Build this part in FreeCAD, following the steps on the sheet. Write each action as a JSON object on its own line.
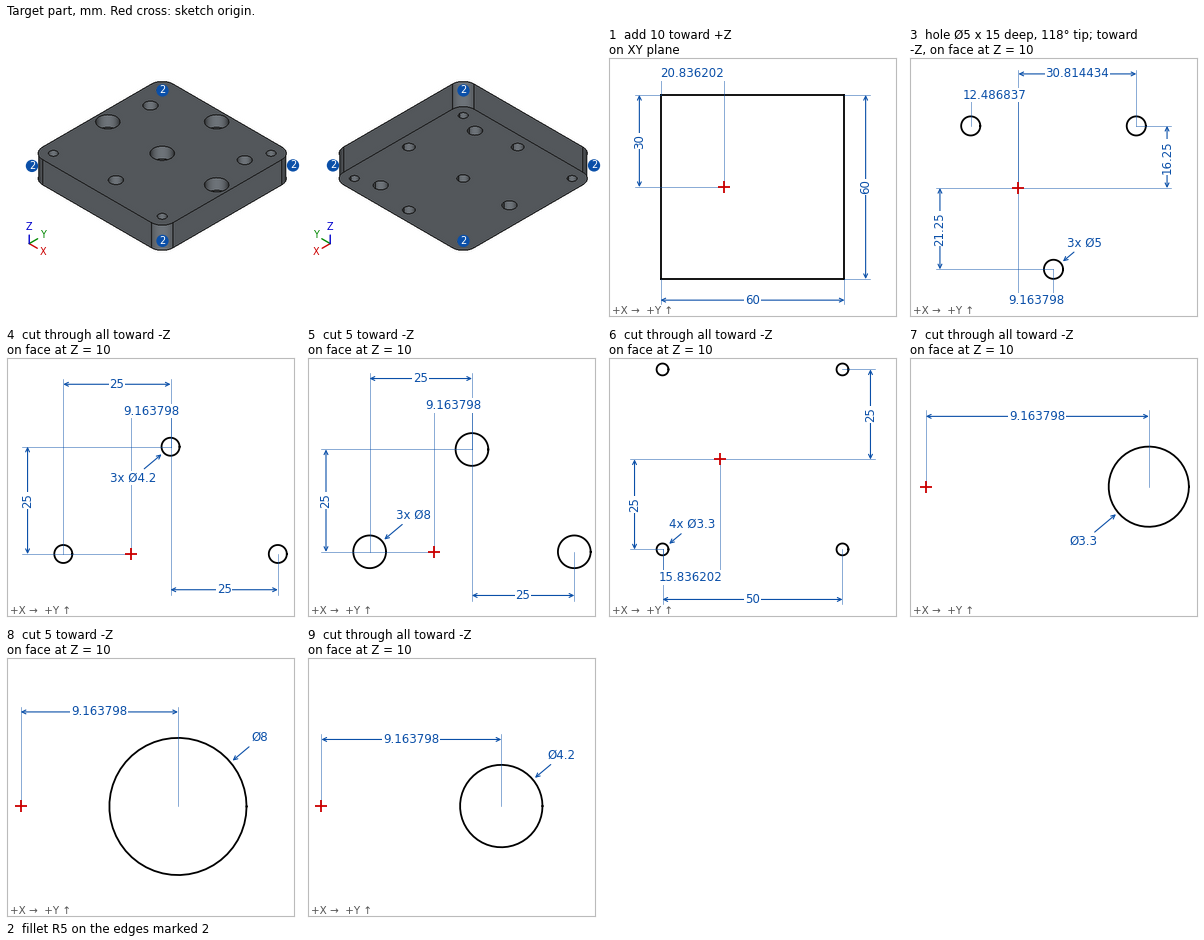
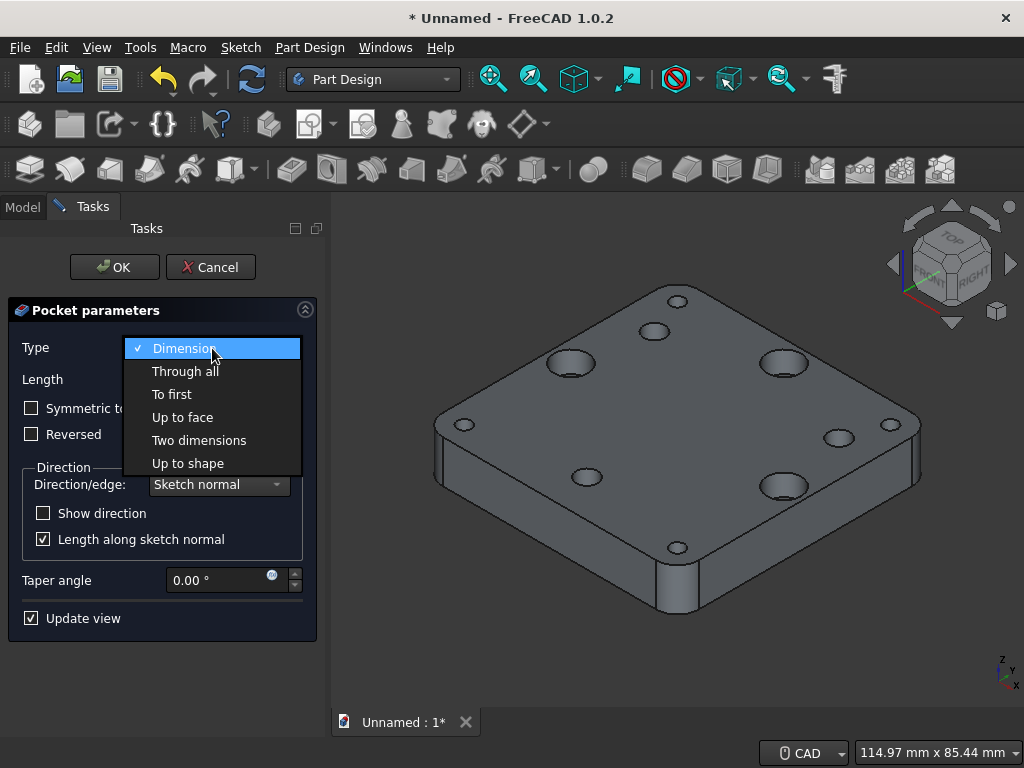
{"action": "left_click", "coordinate": [212, 372]}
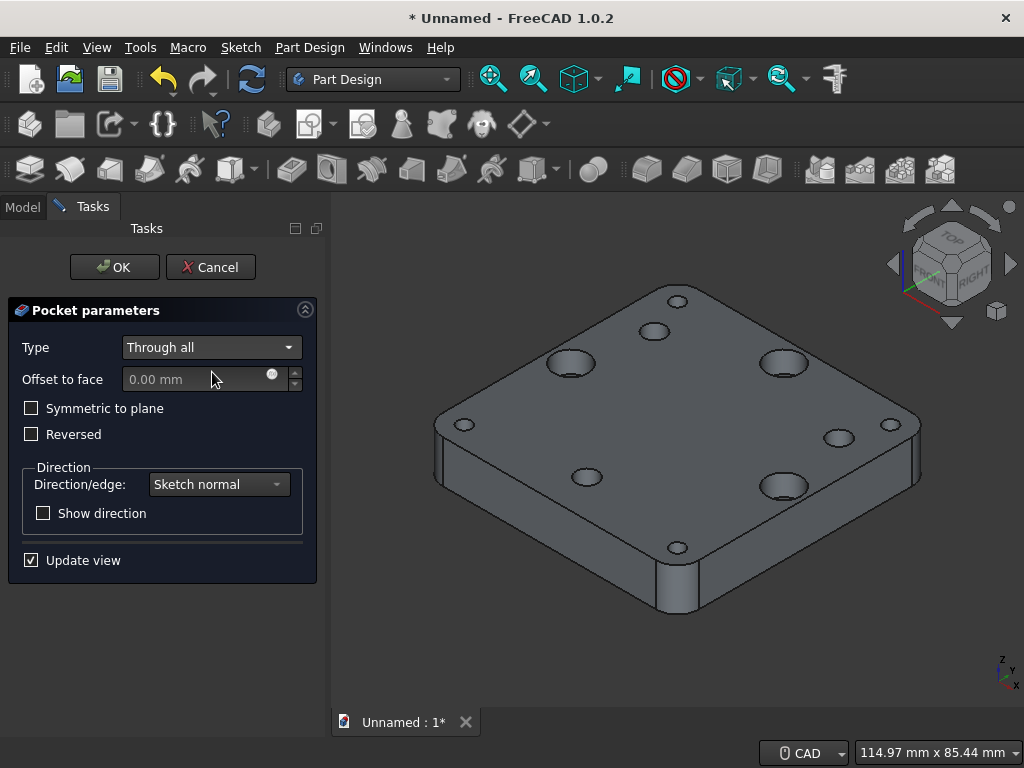
{"action": "left_click", "coordinate": [115, 267]}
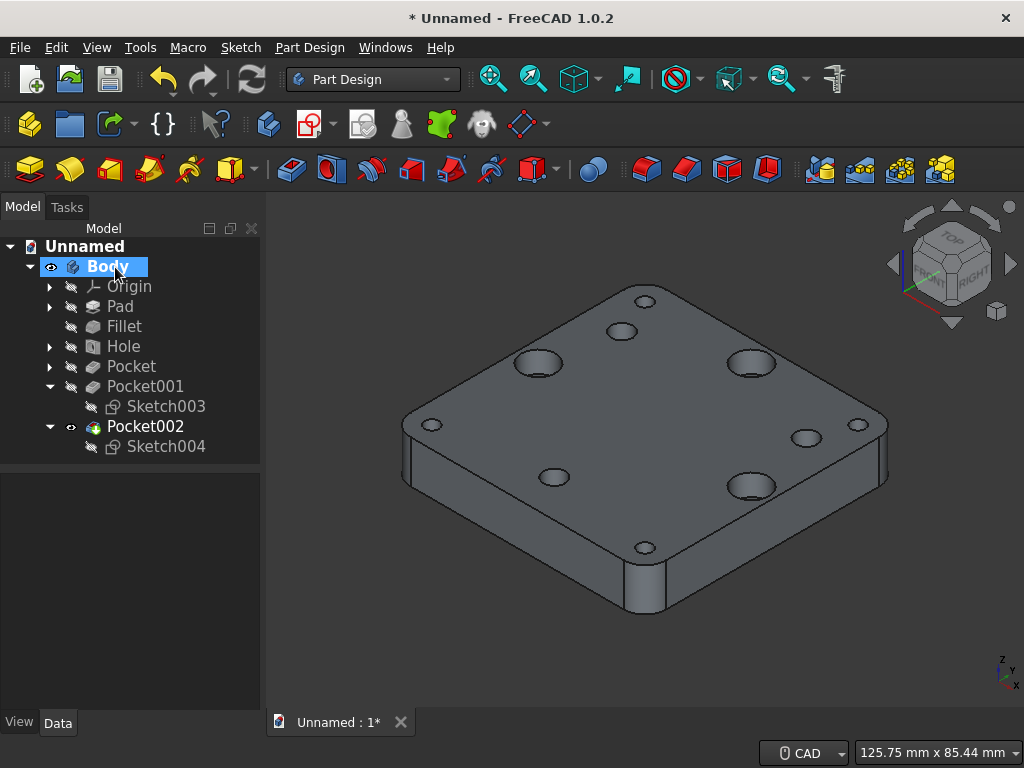
{"action": "left_click", "coordinate": [645, 424]}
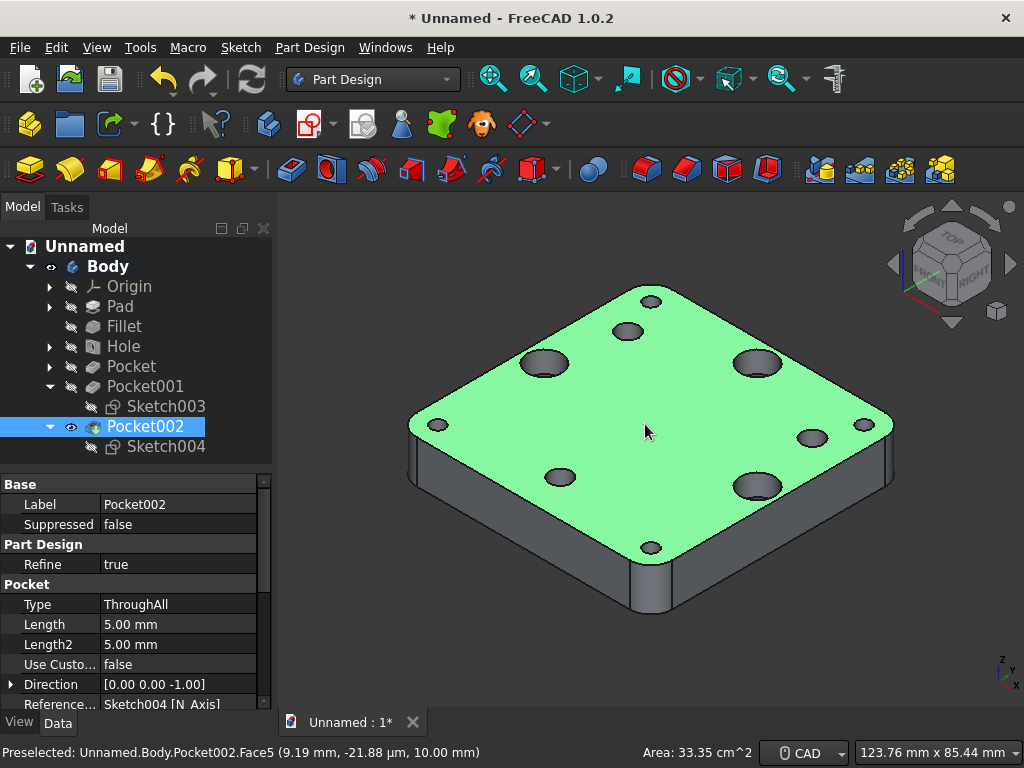
{"action": "left_click", "coordinate": [310, 124]}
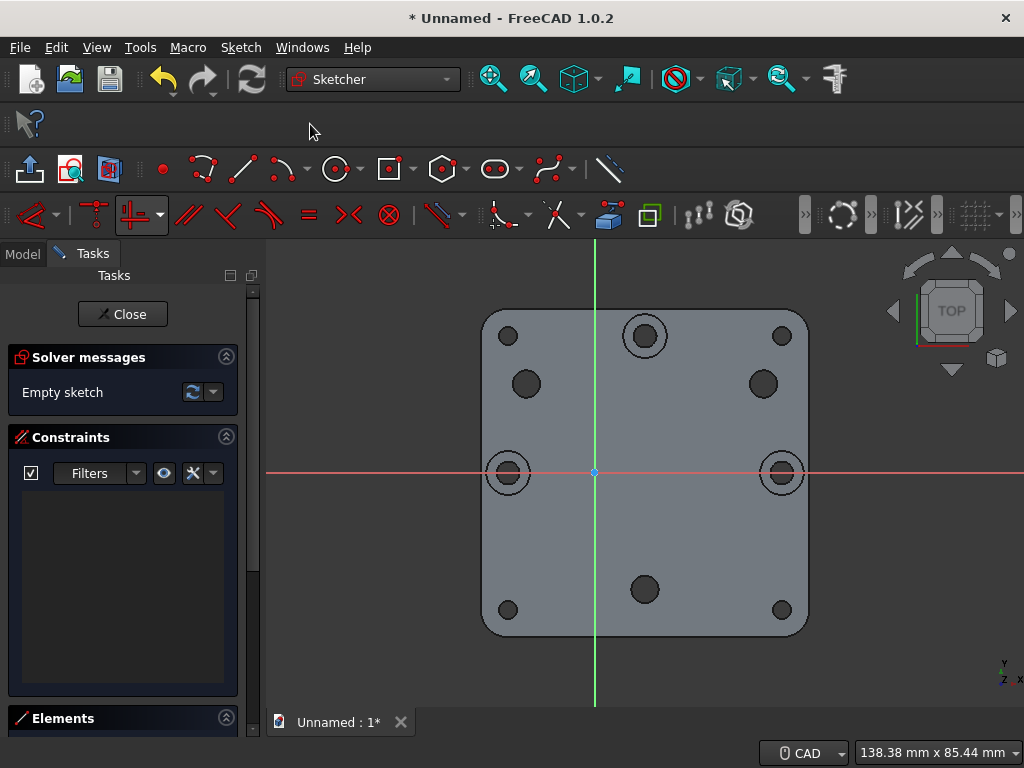
{"action": "scroll", "coordinate": [649, 473], "scroll_direction": "up", "scroll_amount": 14}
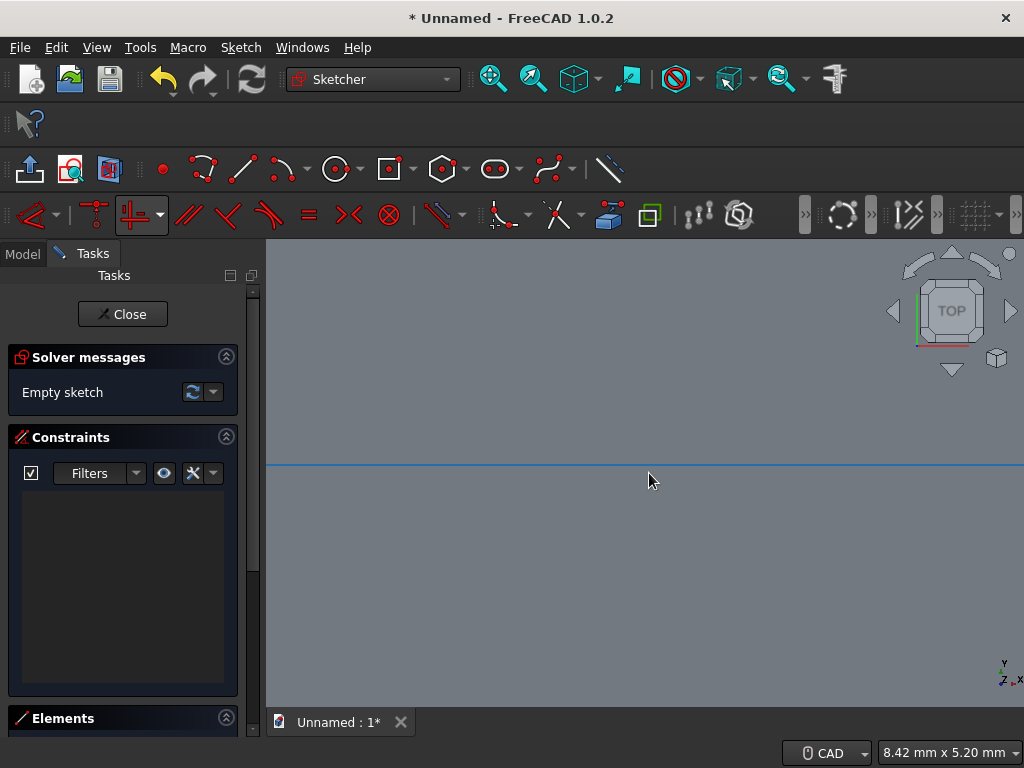
{"action": "left_click", "coordinate": [336, 170]}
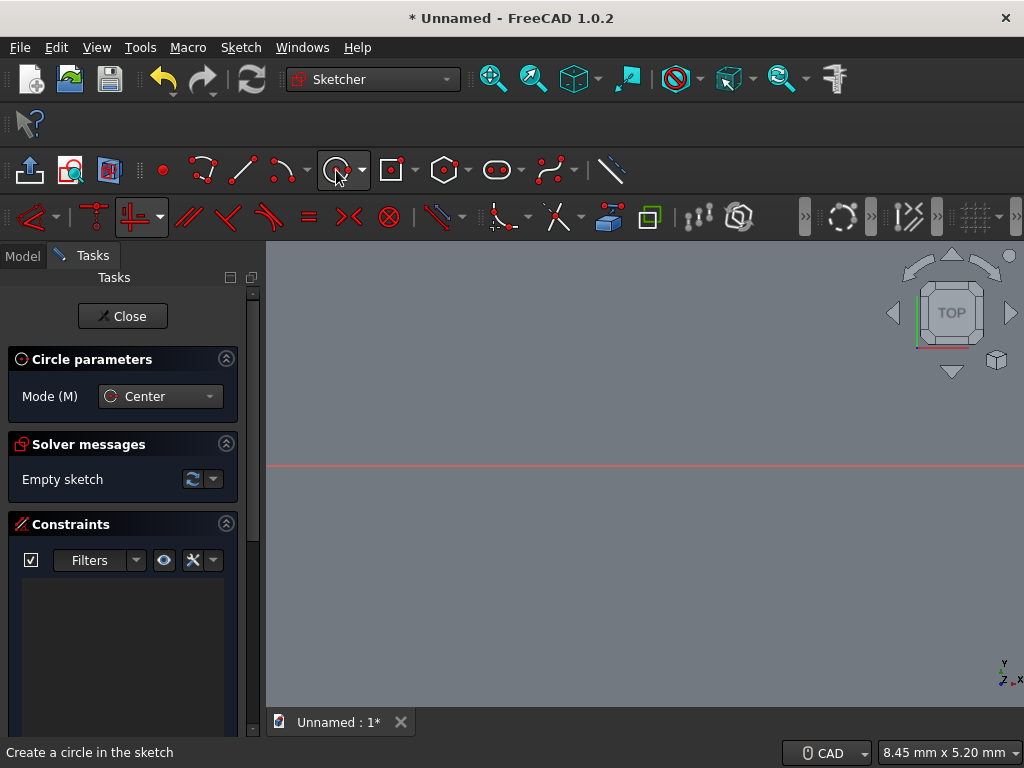
{"action": "left_click", "coordinate": [576, 466]}
{"action": "mouse_move", "coordinate": [680, 362]}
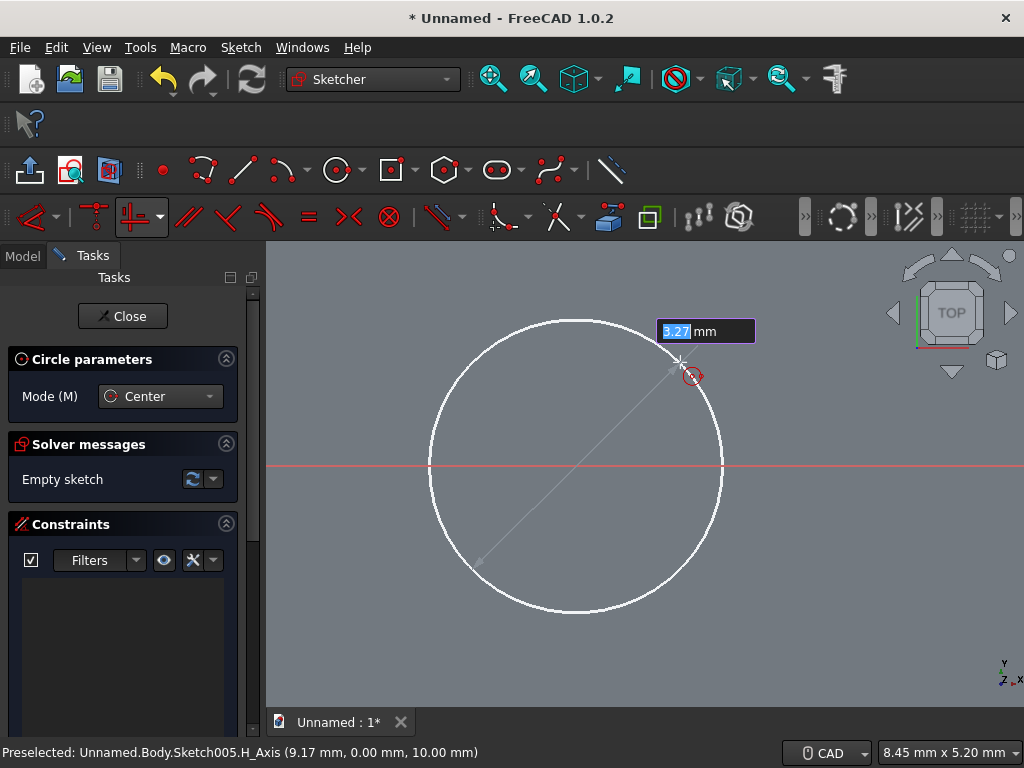
{"action": "type", "text": "3.3"}
{"action": "key", "text": "Return"}
{"action": "key", "text": "Escape"}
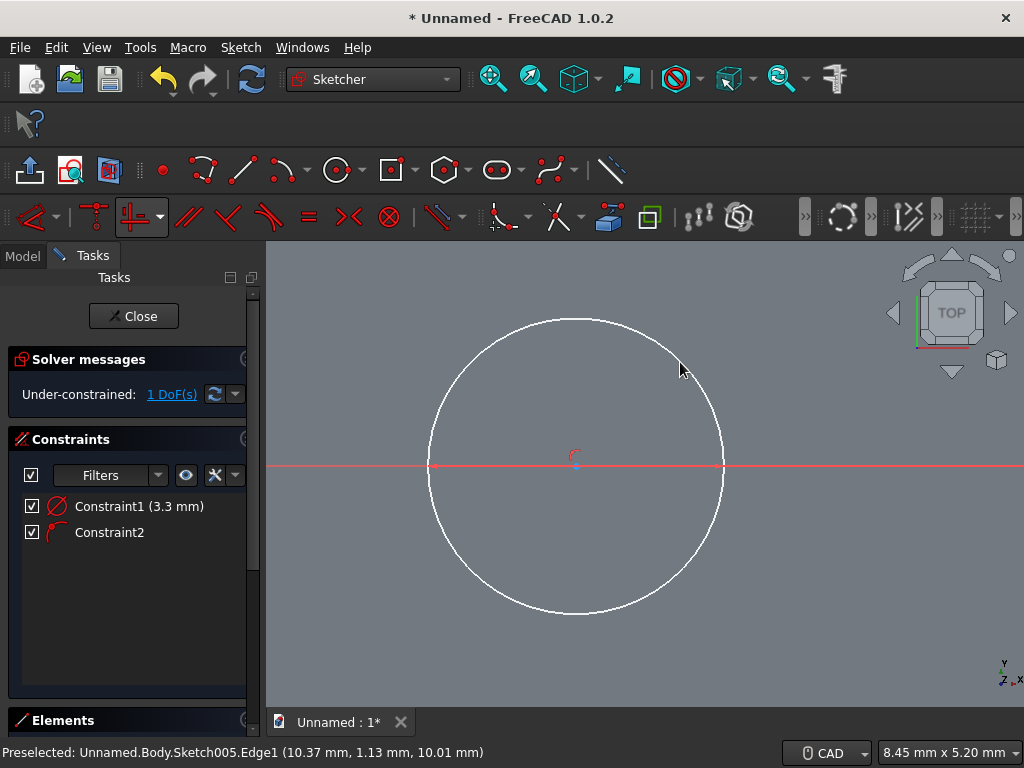
{"action": "left_click", "coordinate": [32, 218]}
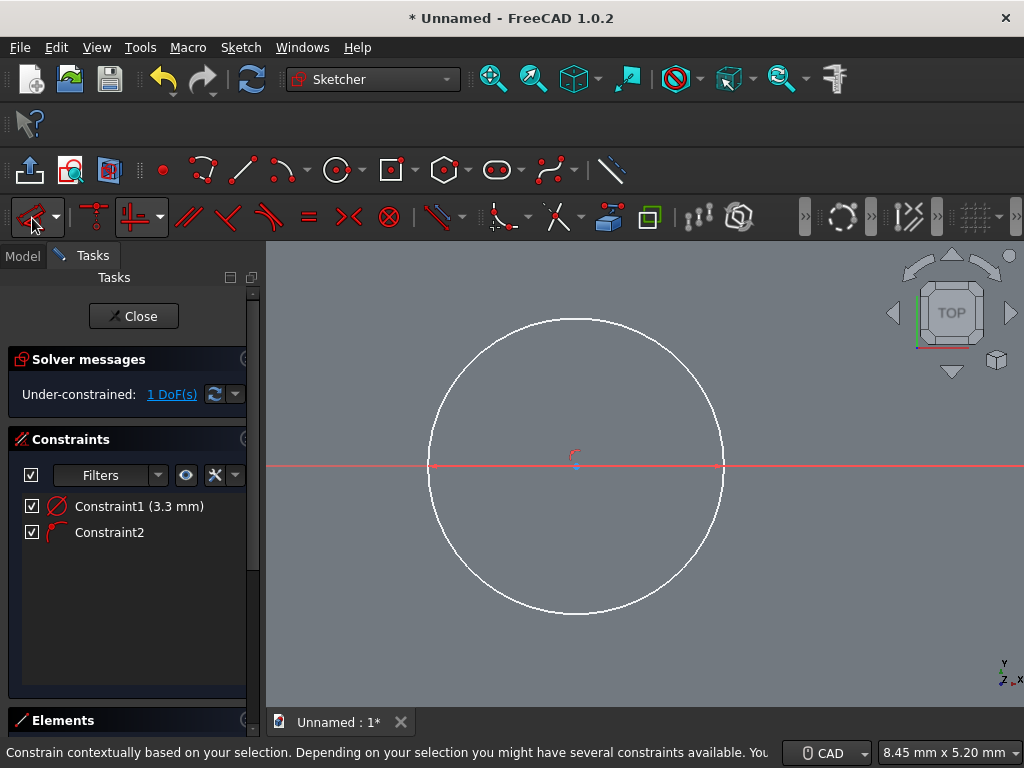
{"action": "left_click", "coordinate": [576, 466]}
{"action": "left_click", "coordinate": [370, 500]}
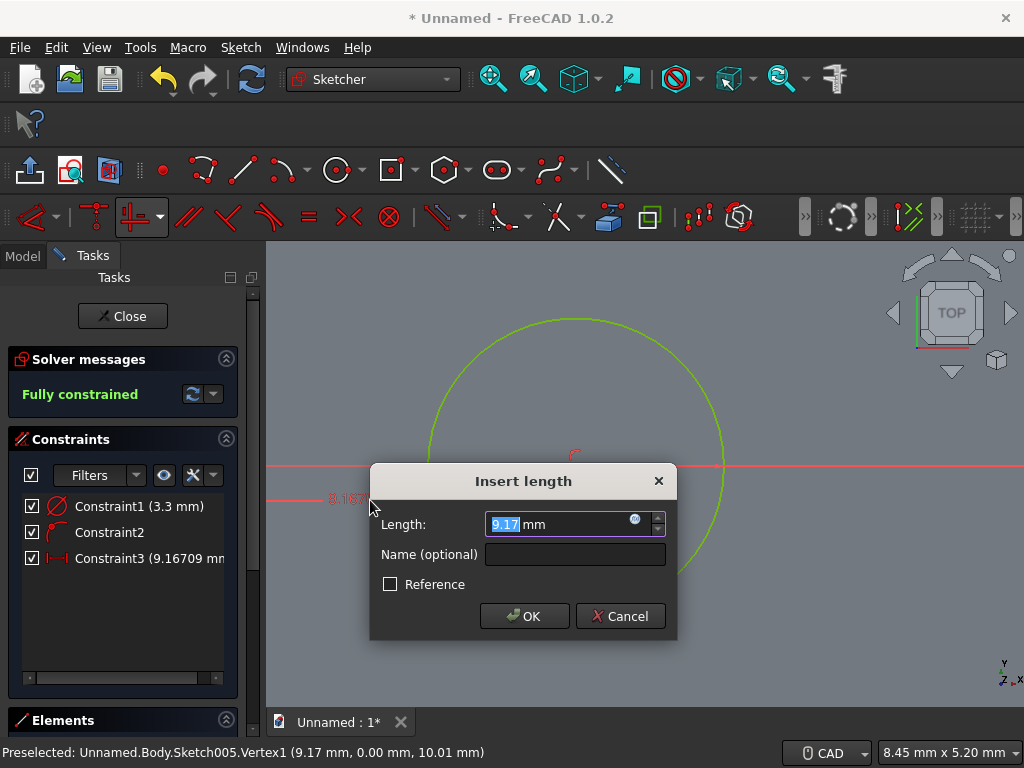
{"action": "type", "text": "9.163798"}
{"action": "key", "text": "Return"}
{"action": "key", "text": "Escape"}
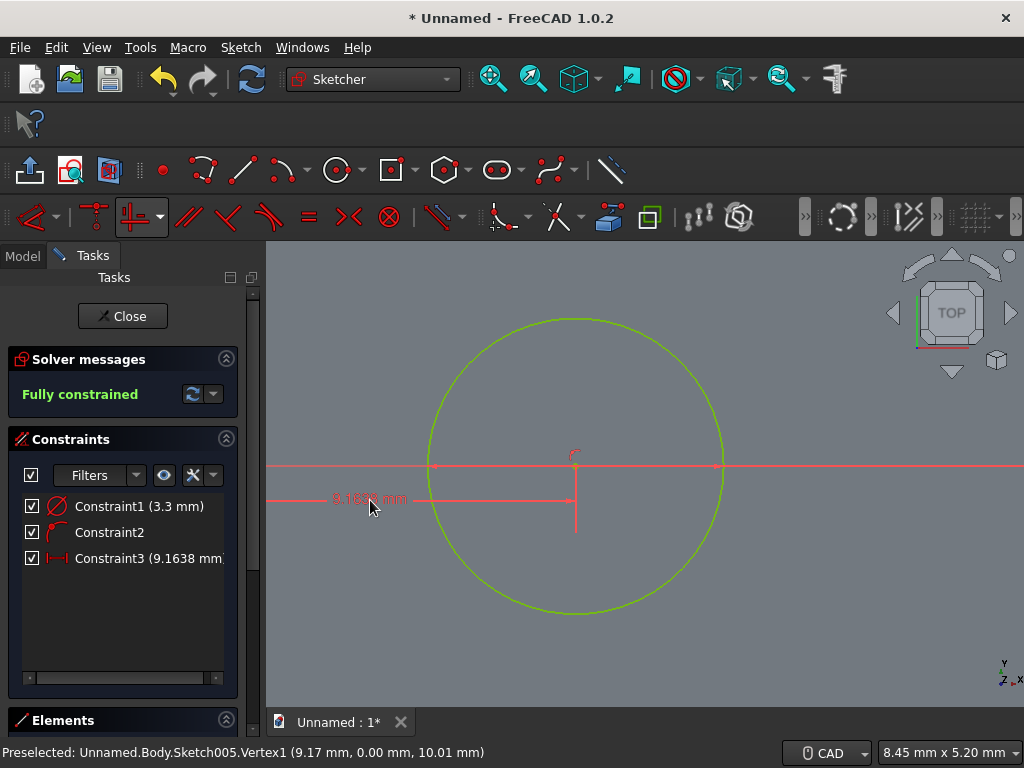
{"action": "left_click", "coordinate": [123, 316]}